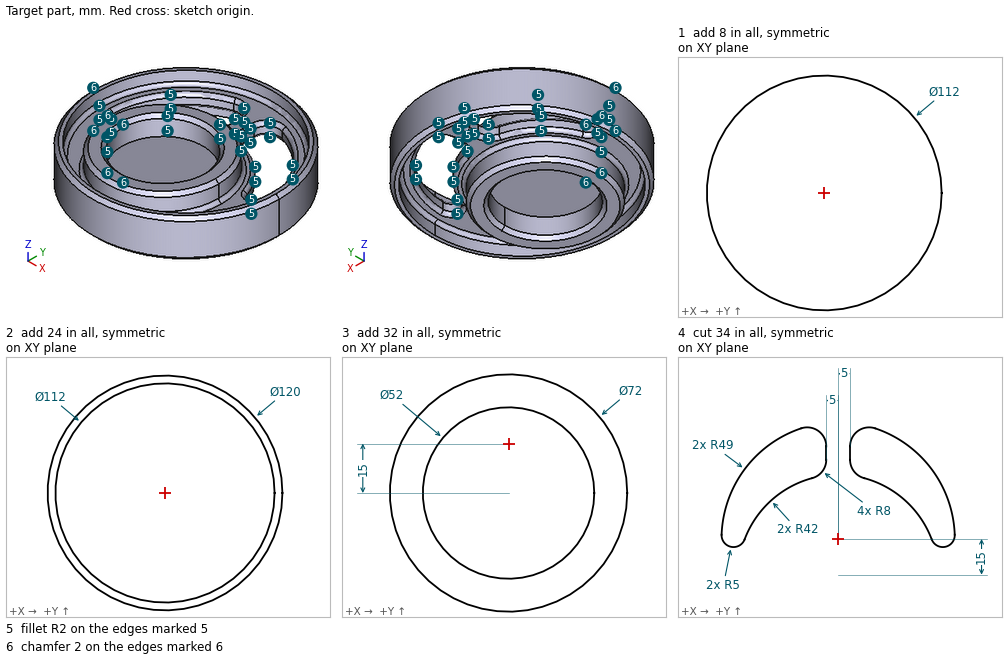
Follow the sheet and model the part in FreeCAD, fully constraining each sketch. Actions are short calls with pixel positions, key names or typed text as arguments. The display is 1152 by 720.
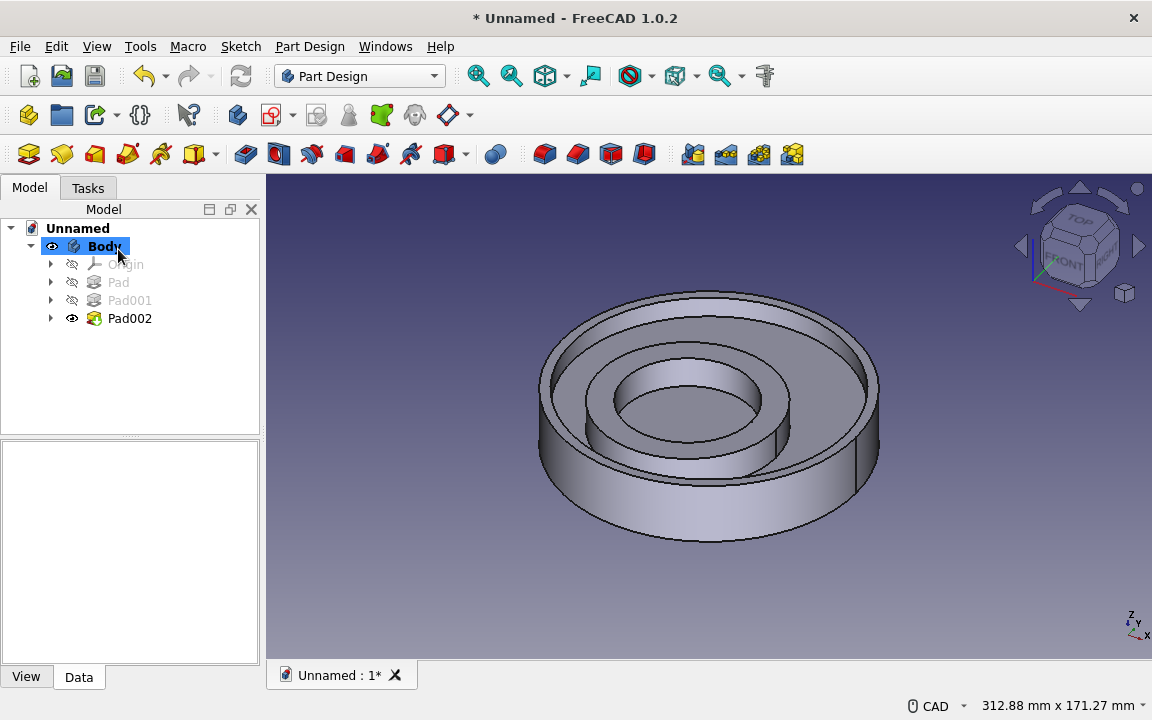
click(270, 116)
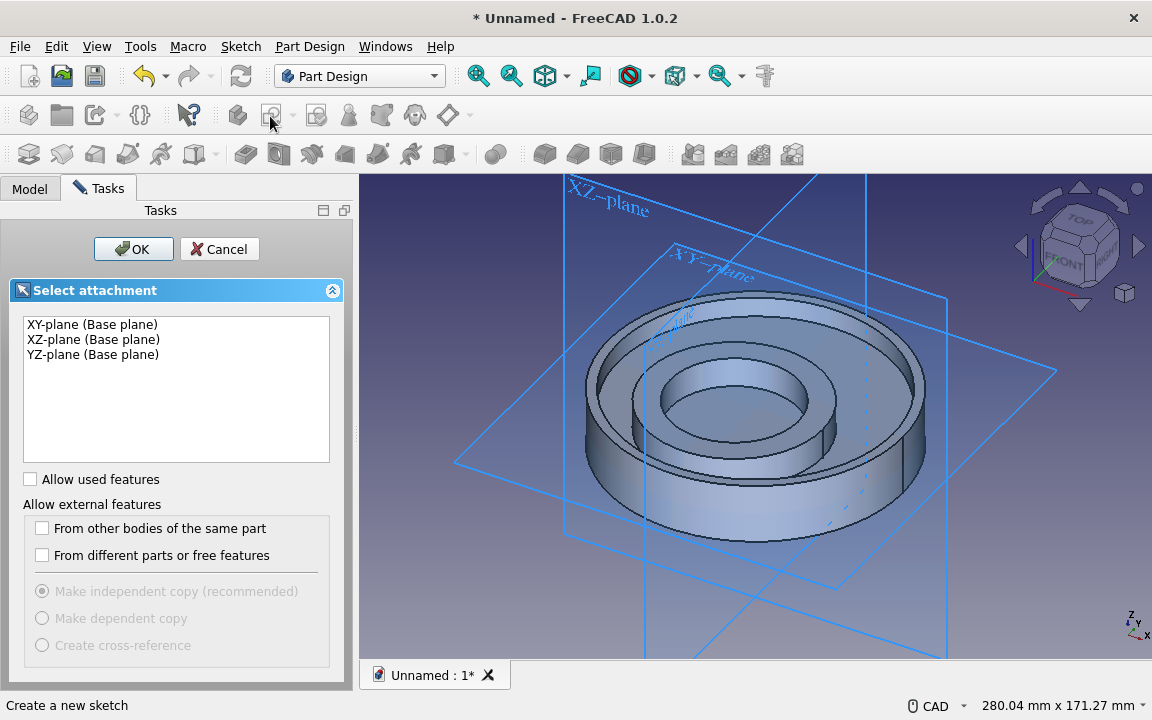
click(84, 324)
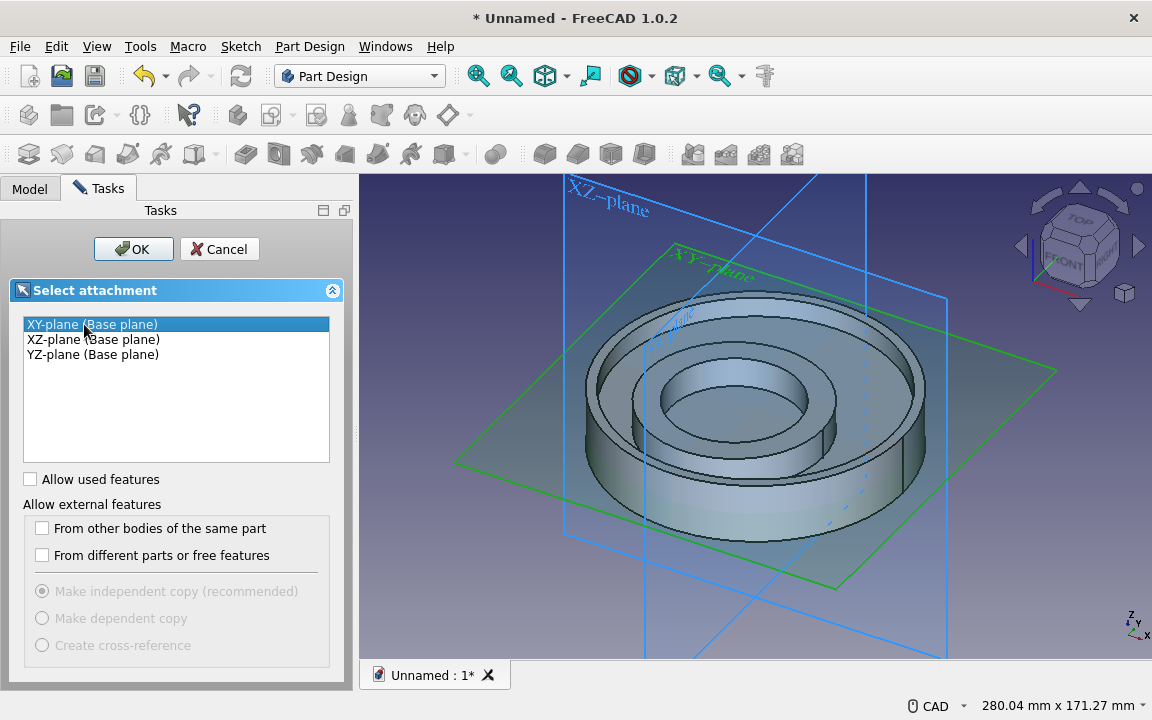
click(134, 249)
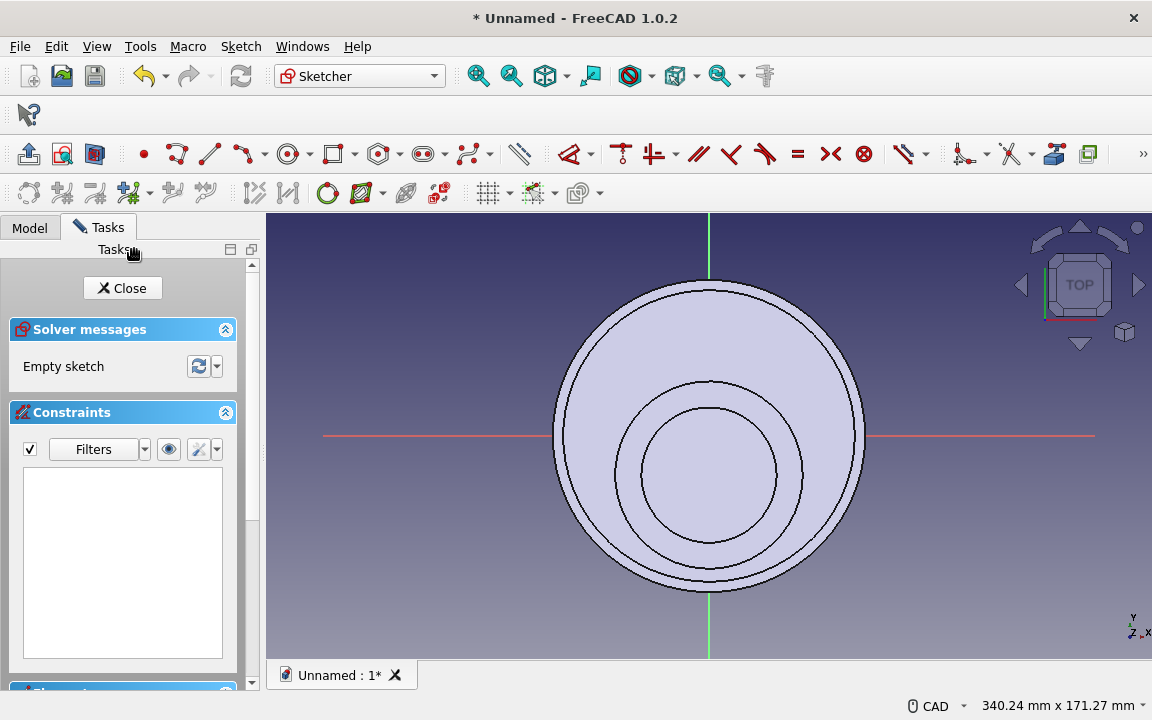
key(q)
key(s)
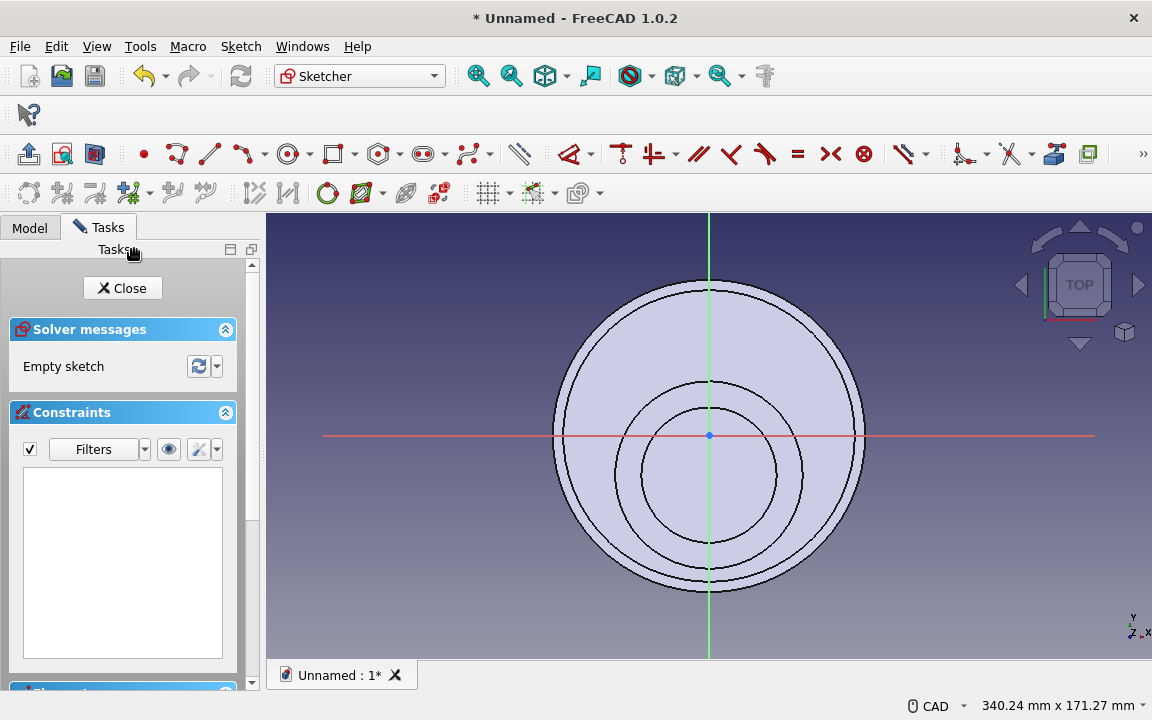
scroll(792, 311, up, 3)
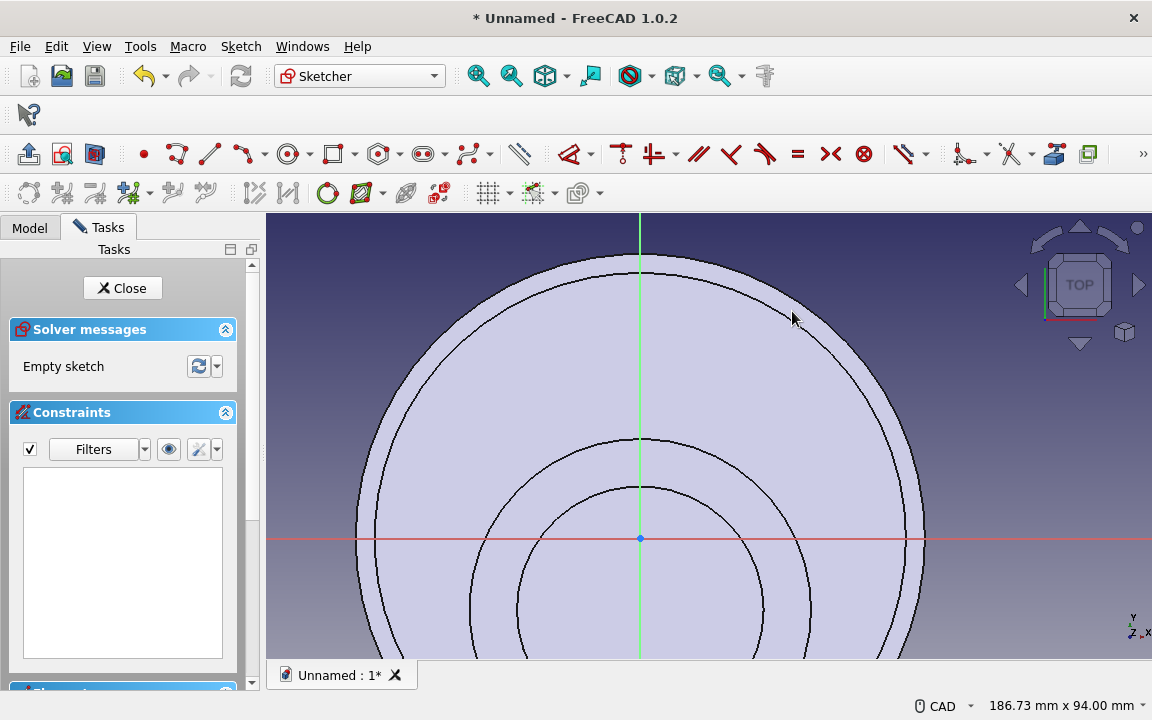
click(210, 154)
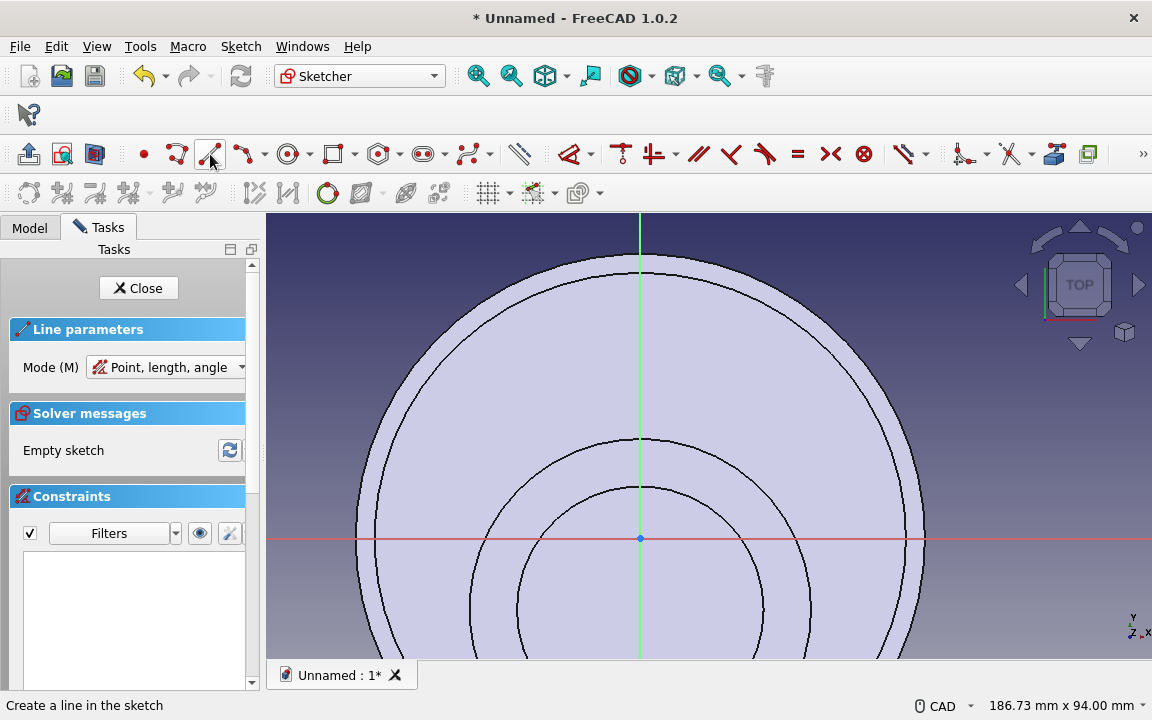
click(617, 381)
click(617, 354)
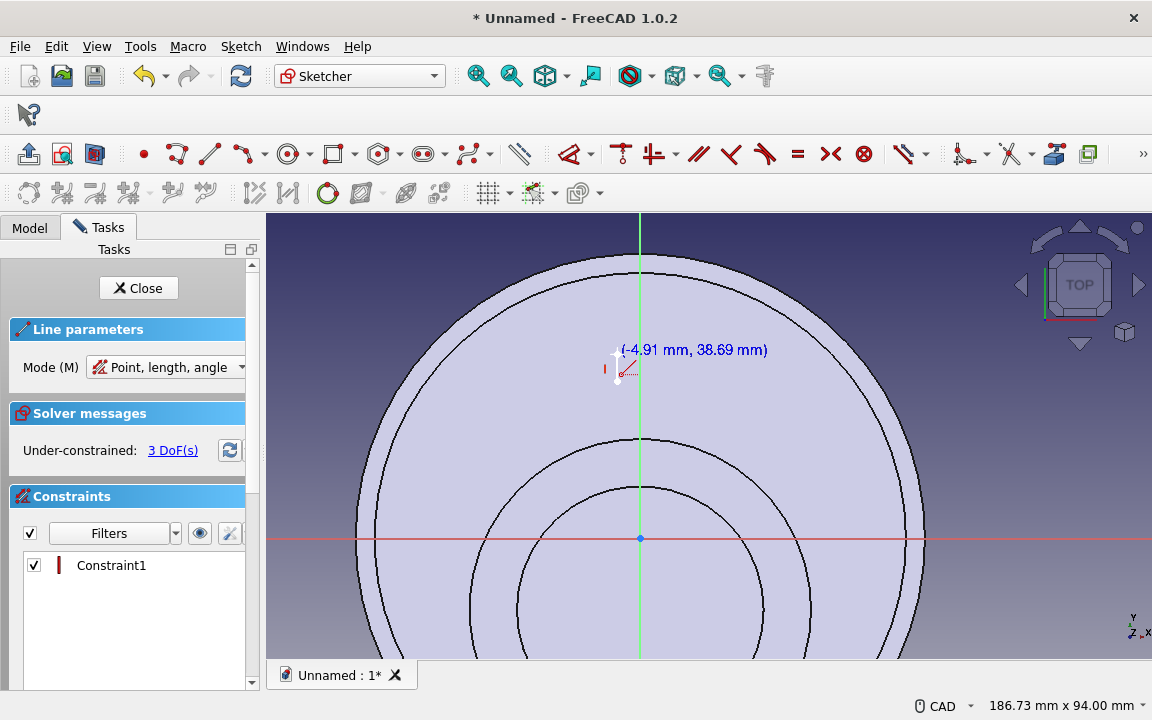
key(g)
key(3)
key(a)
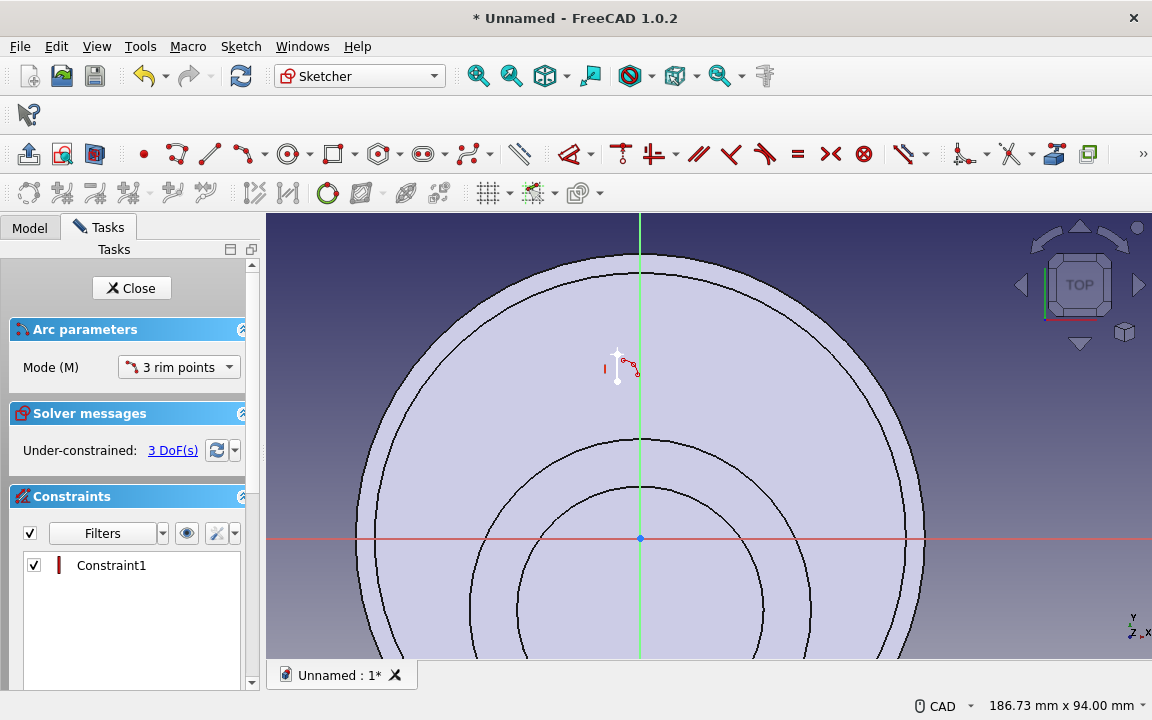
click(617, 355)
click(567, 318)
click(601, 323)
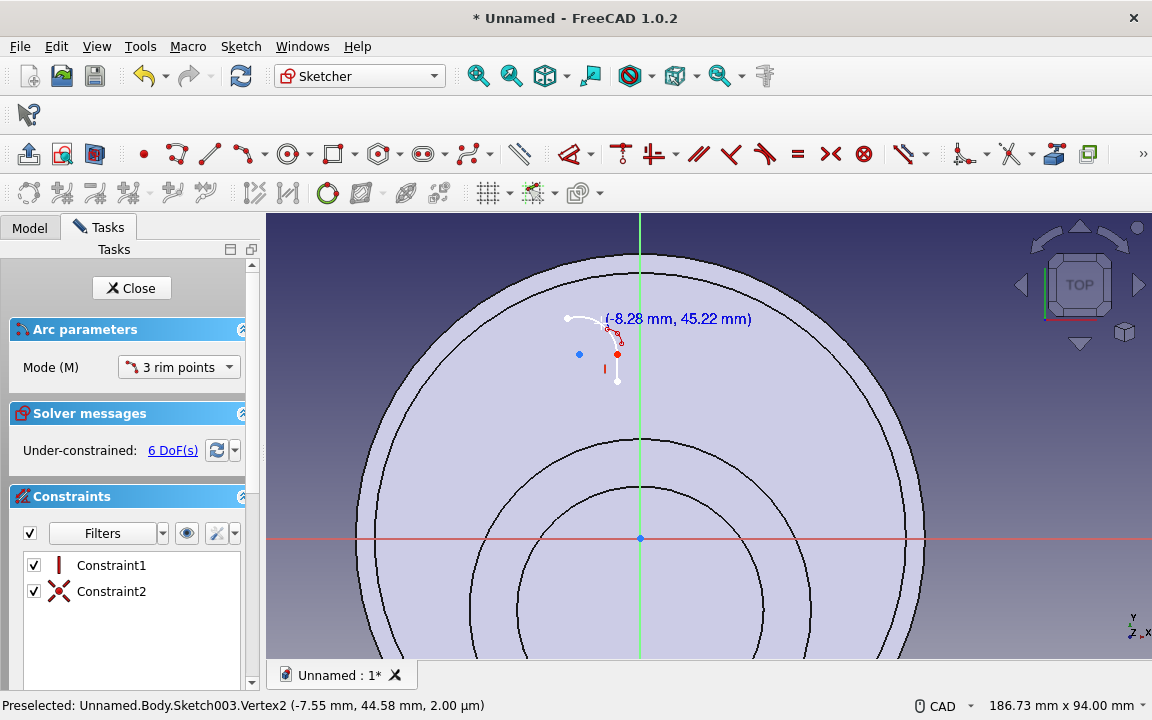
click(567, 319)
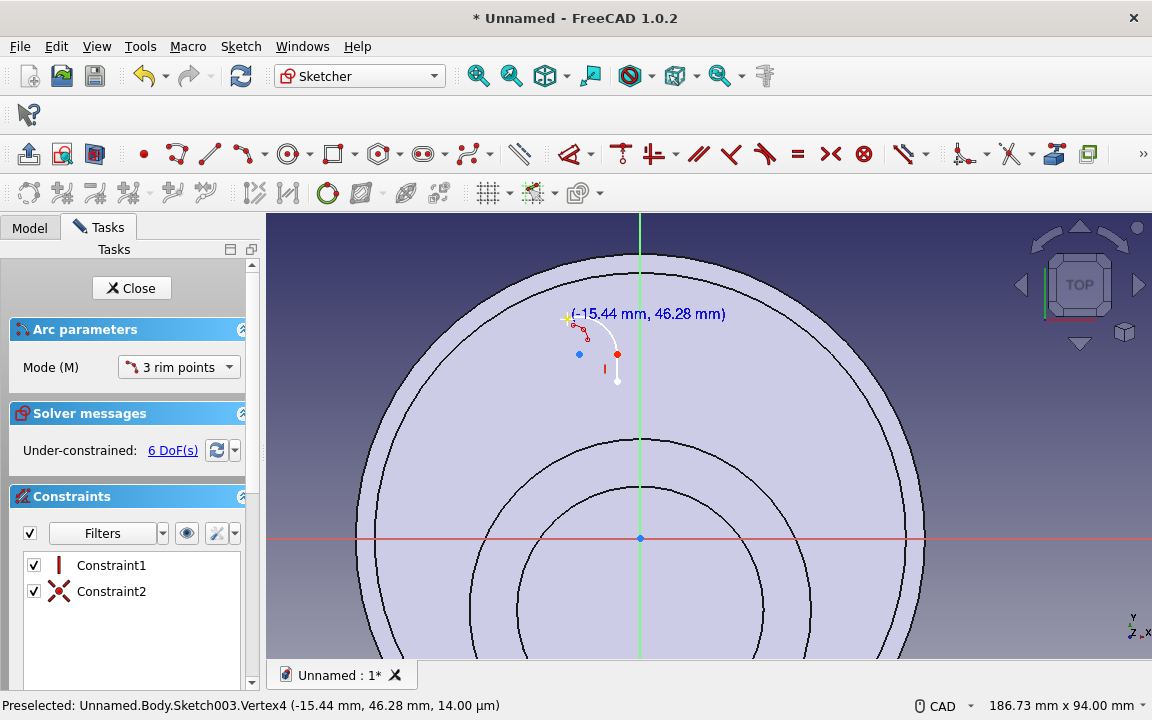
scroll(408, 530, up, 4)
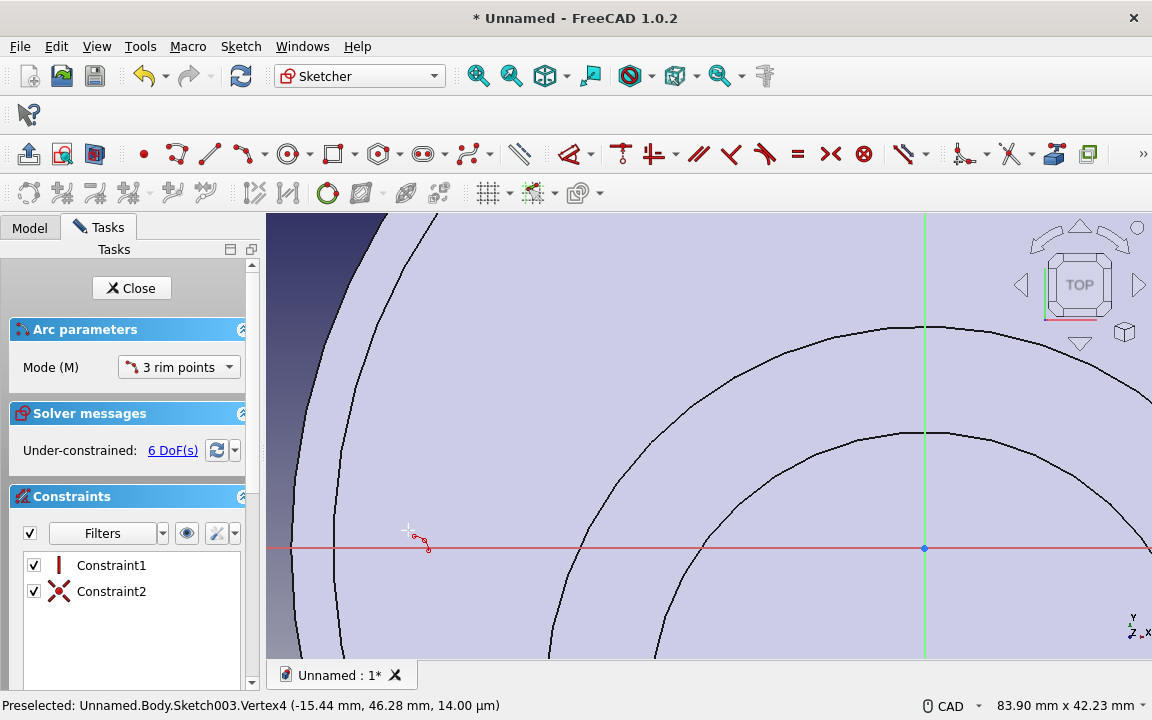
click(408, 529)